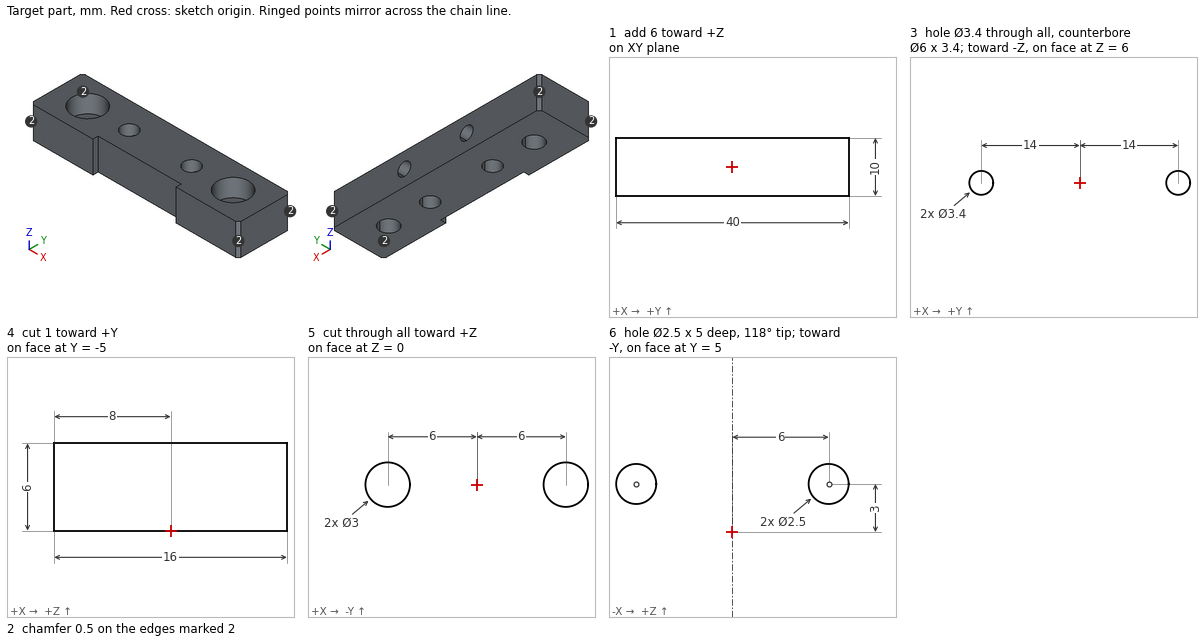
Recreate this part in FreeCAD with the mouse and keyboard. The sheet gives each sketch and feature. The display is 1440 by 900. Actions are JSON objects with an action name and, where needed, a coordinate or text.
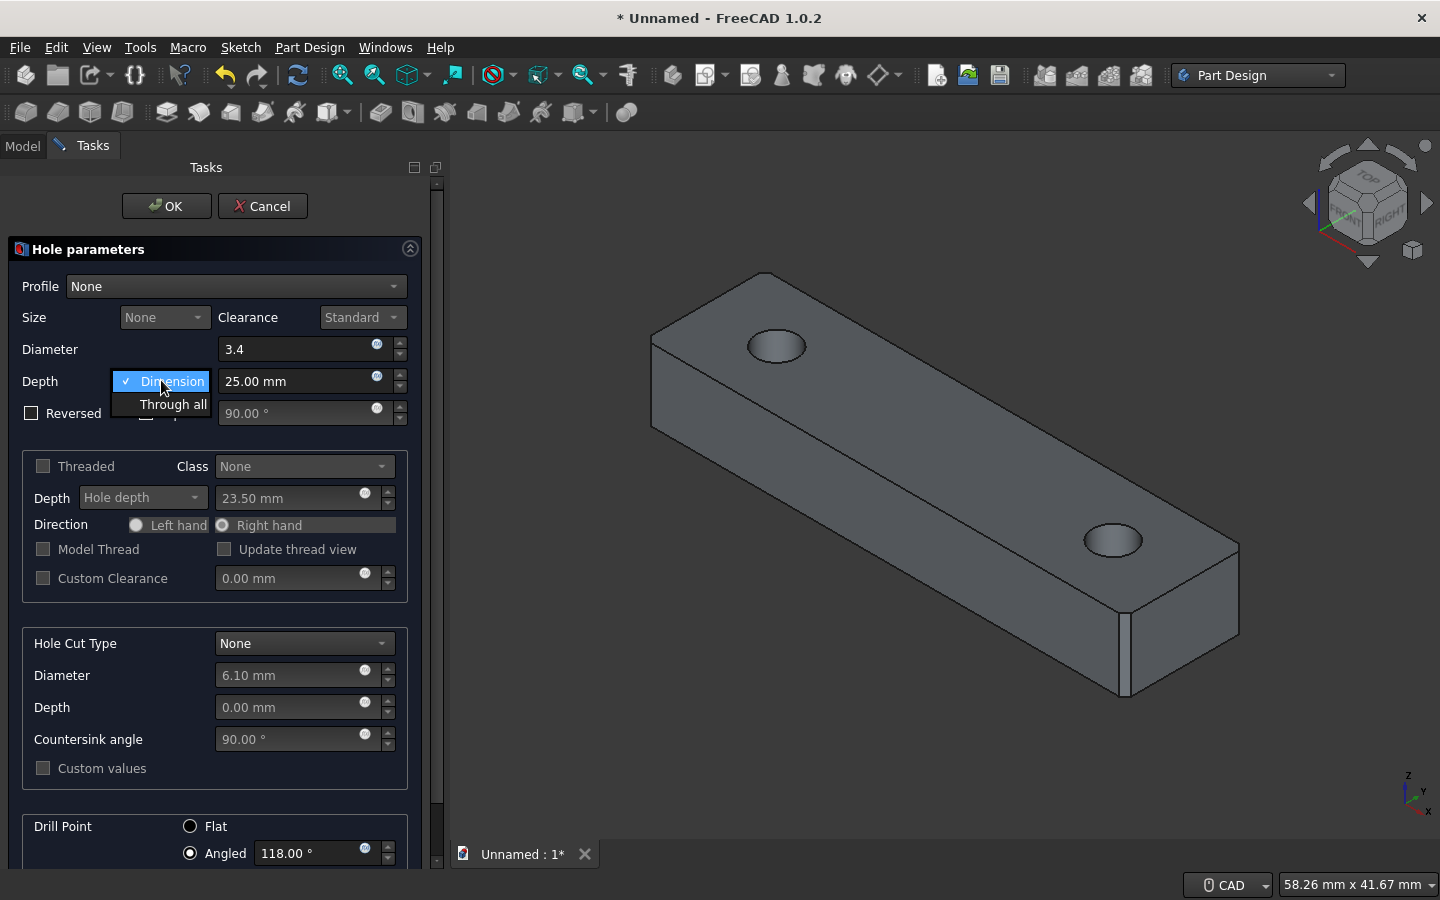
{"action": "left_click", "coordinate": [160, 404]}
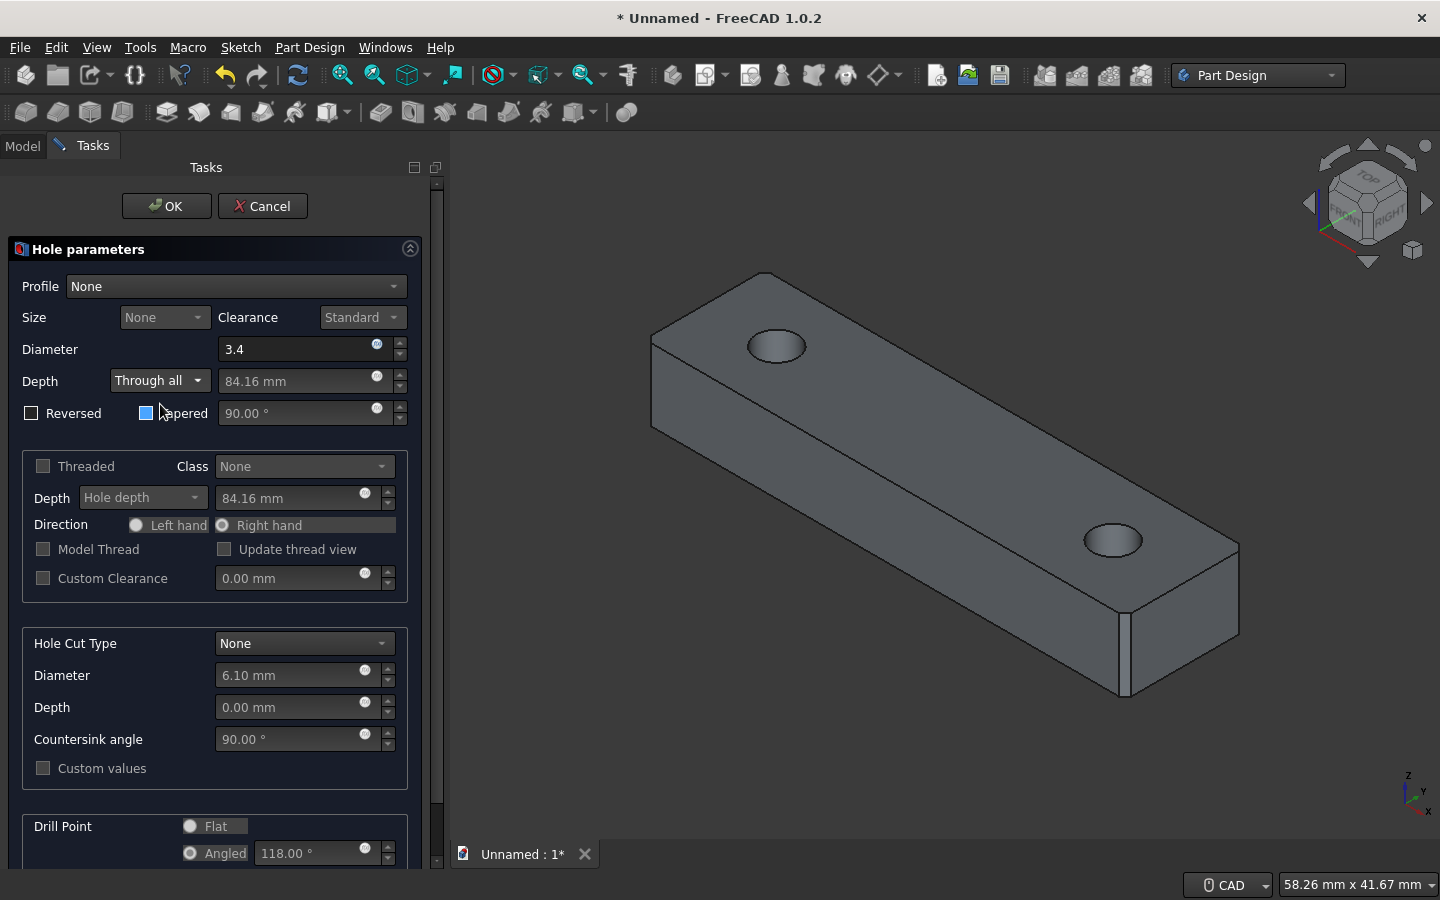
{"action": "left_click", "coordinate": [306, 644]}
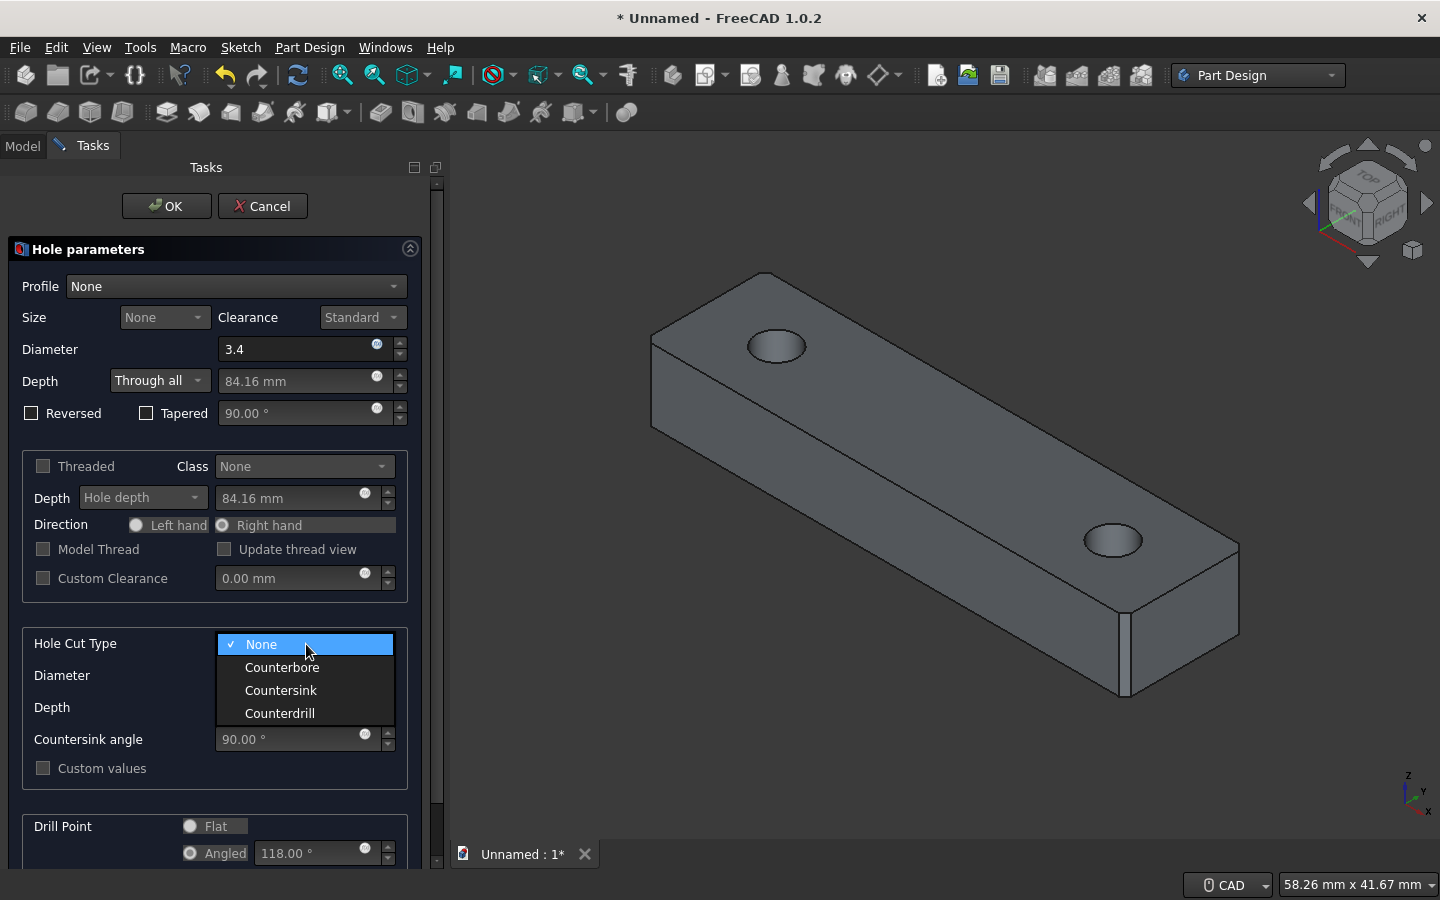
{"action": "left_click", "coordinate": [304, 668]}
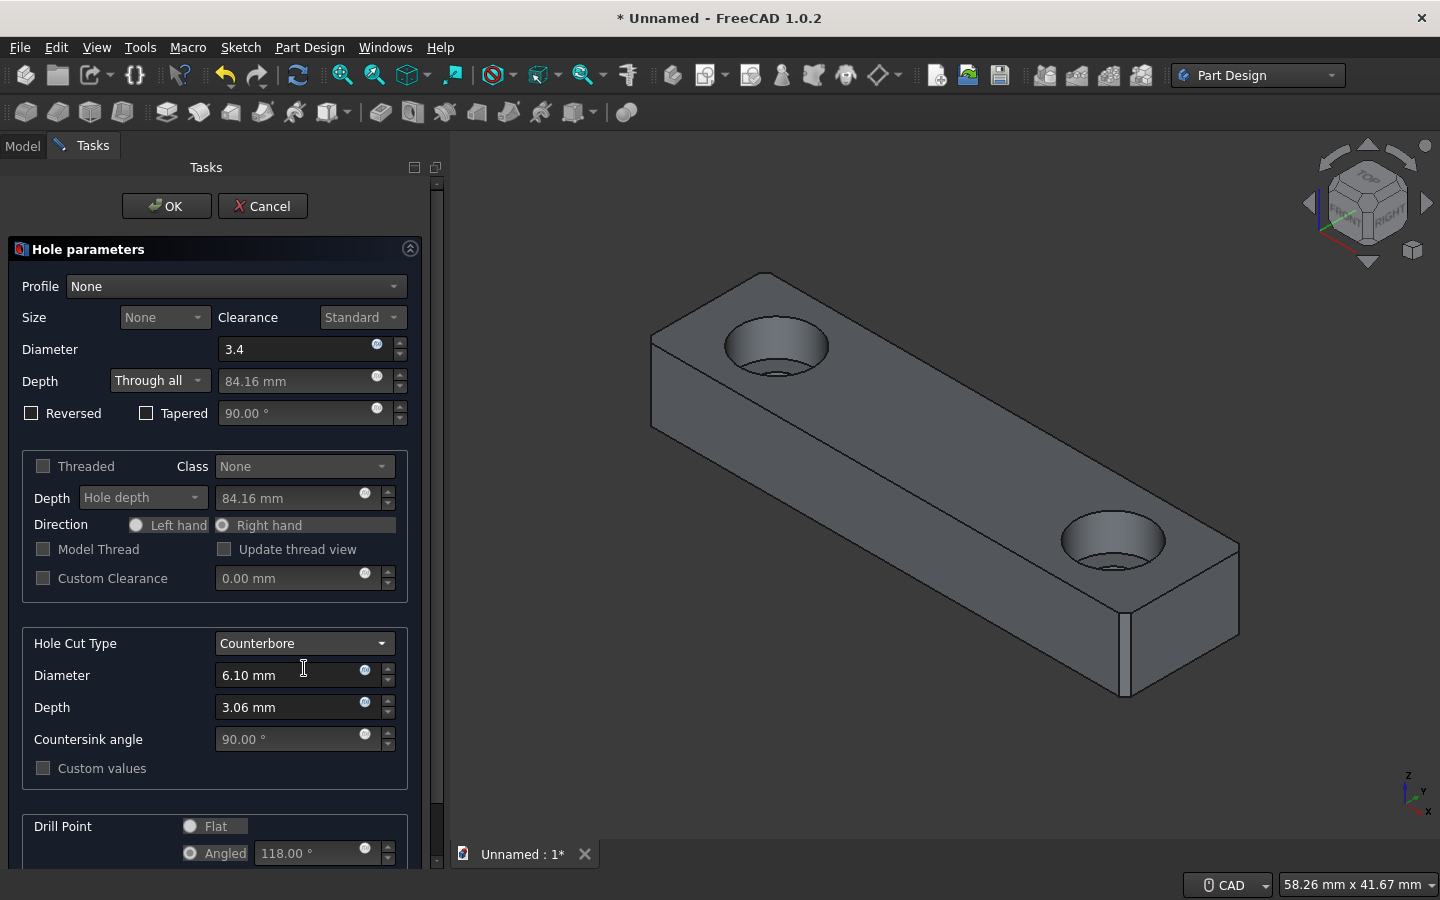
{"action": "triple_click", "coordinate": [298, 675]}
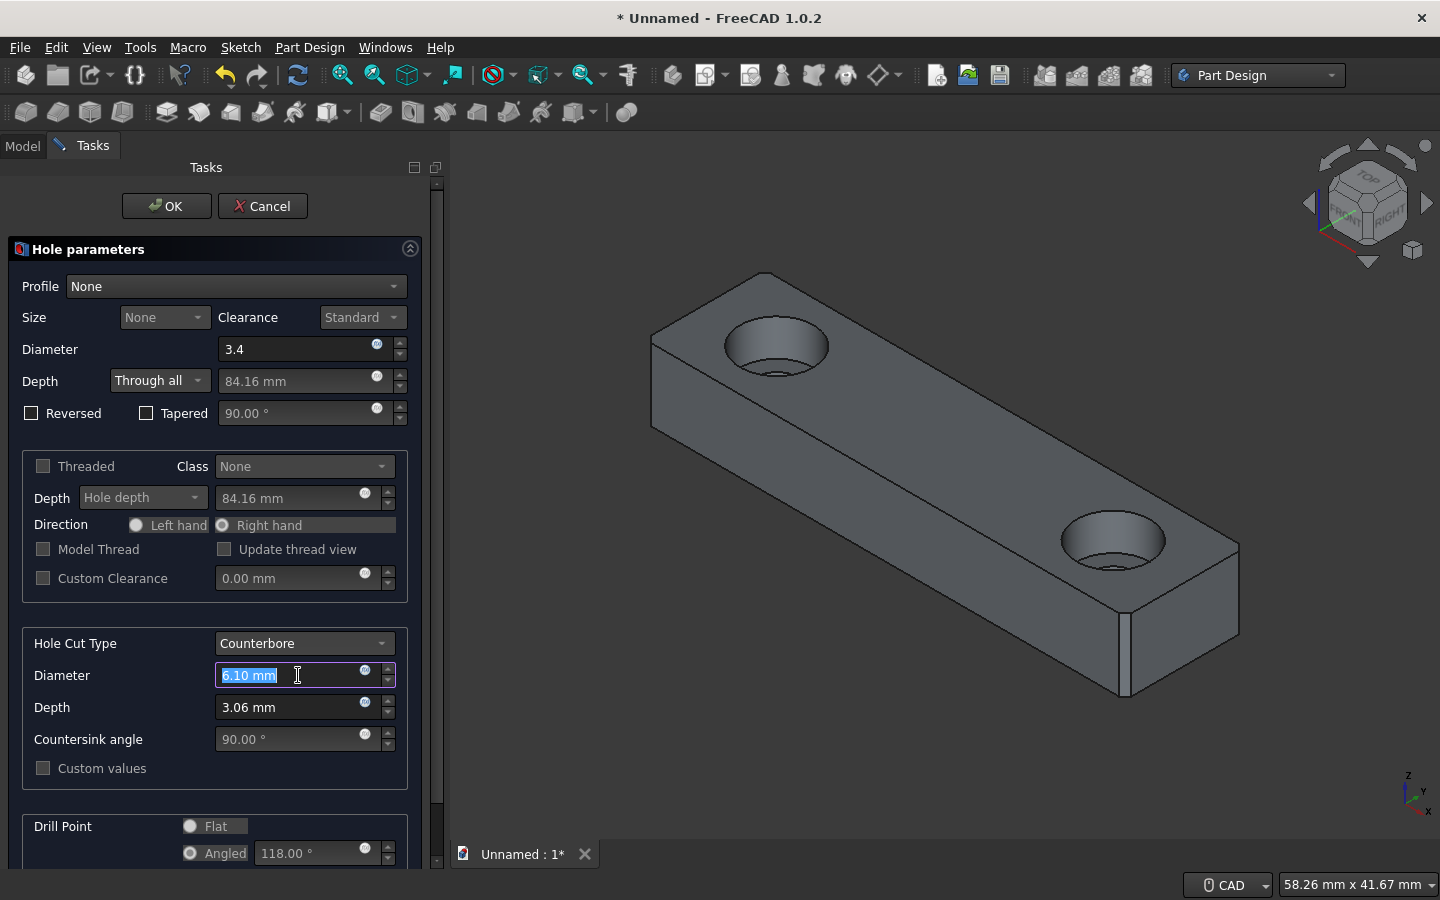
{"action": "type", "text": "6"}
{"action": "key", "text": "Tab"}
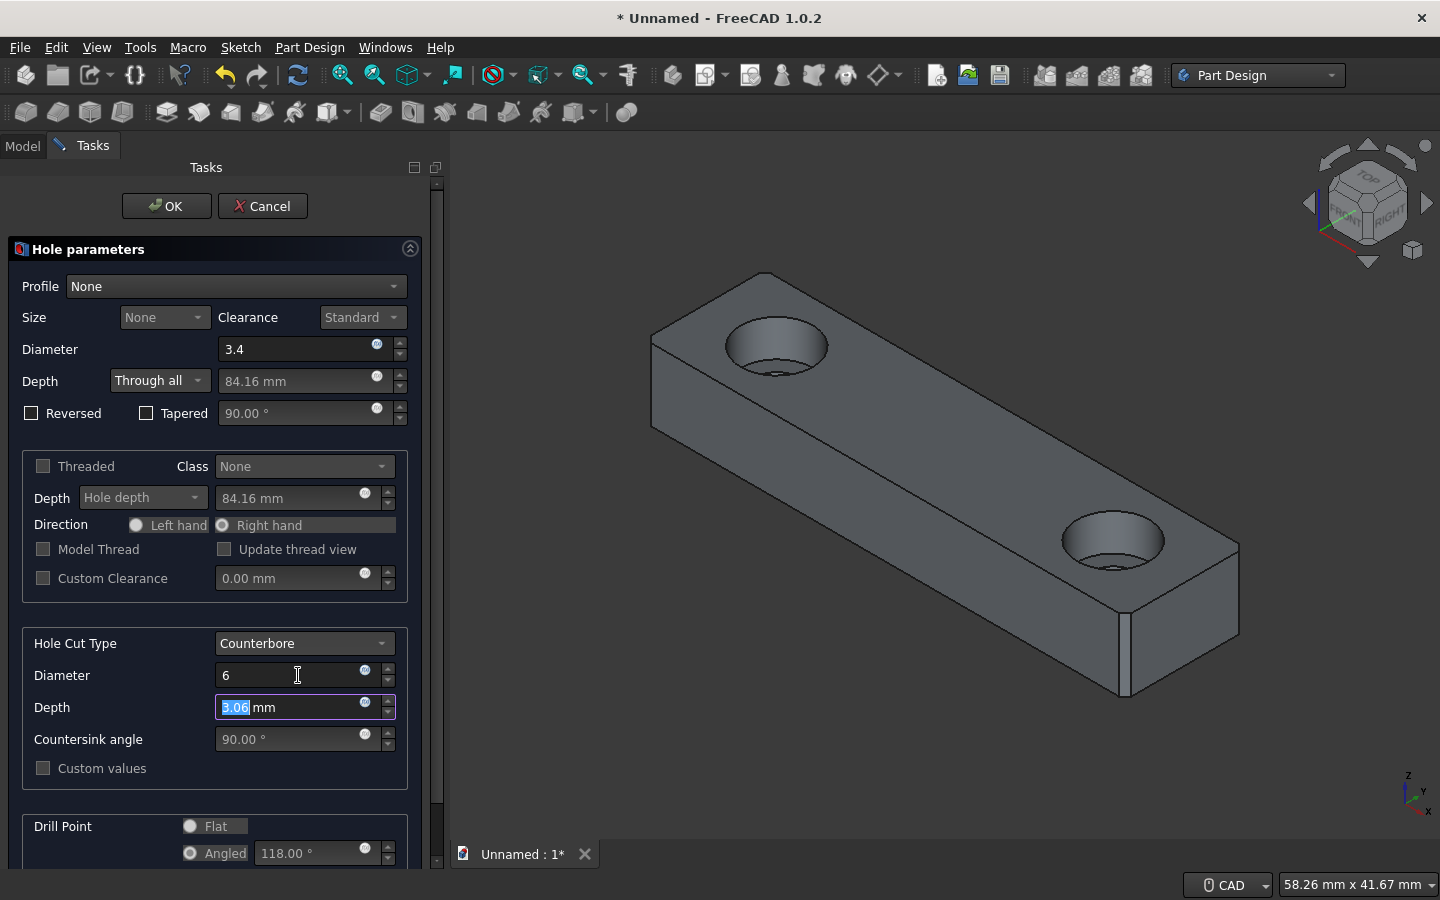
{"action": "type", "text": "3.4"}
{"action": "key", "text": "Tab"}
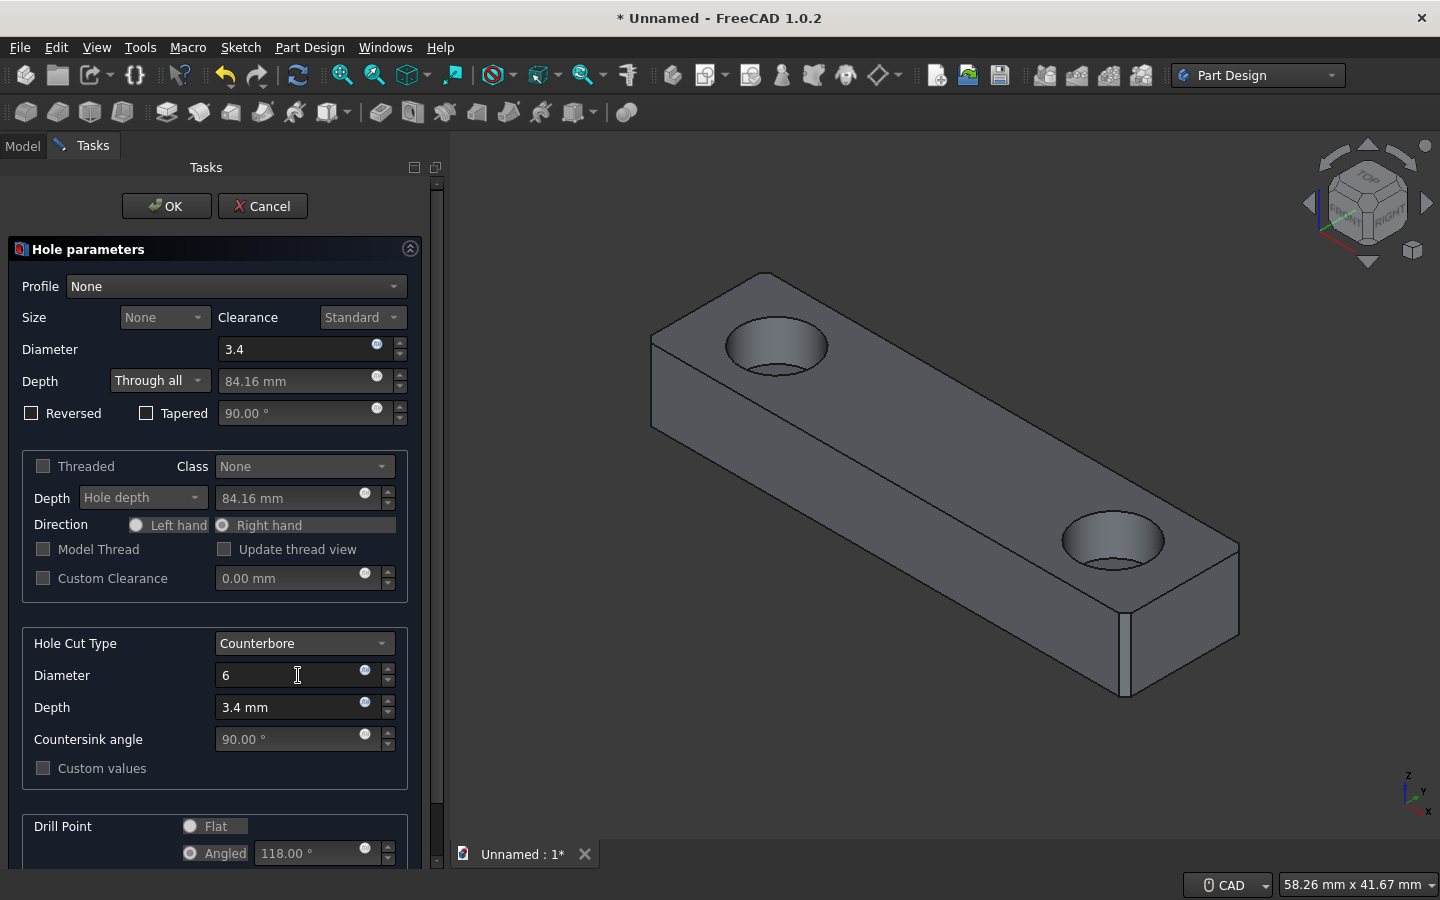
{"action": "left_click", "coordinate": [167, 206]}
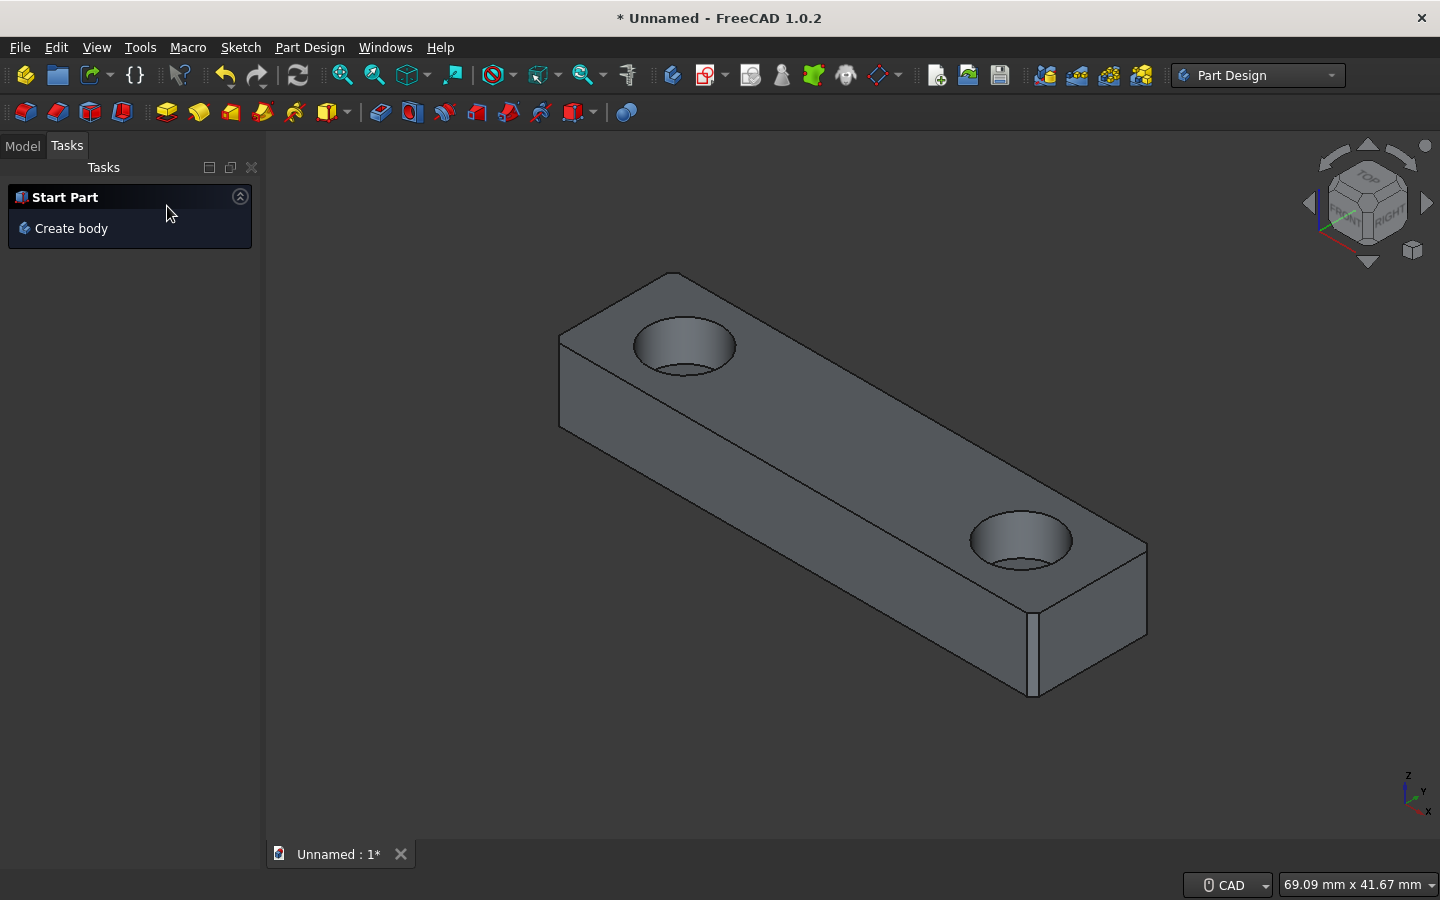
{"action": "left_click", "coordinate": [927, 596]}